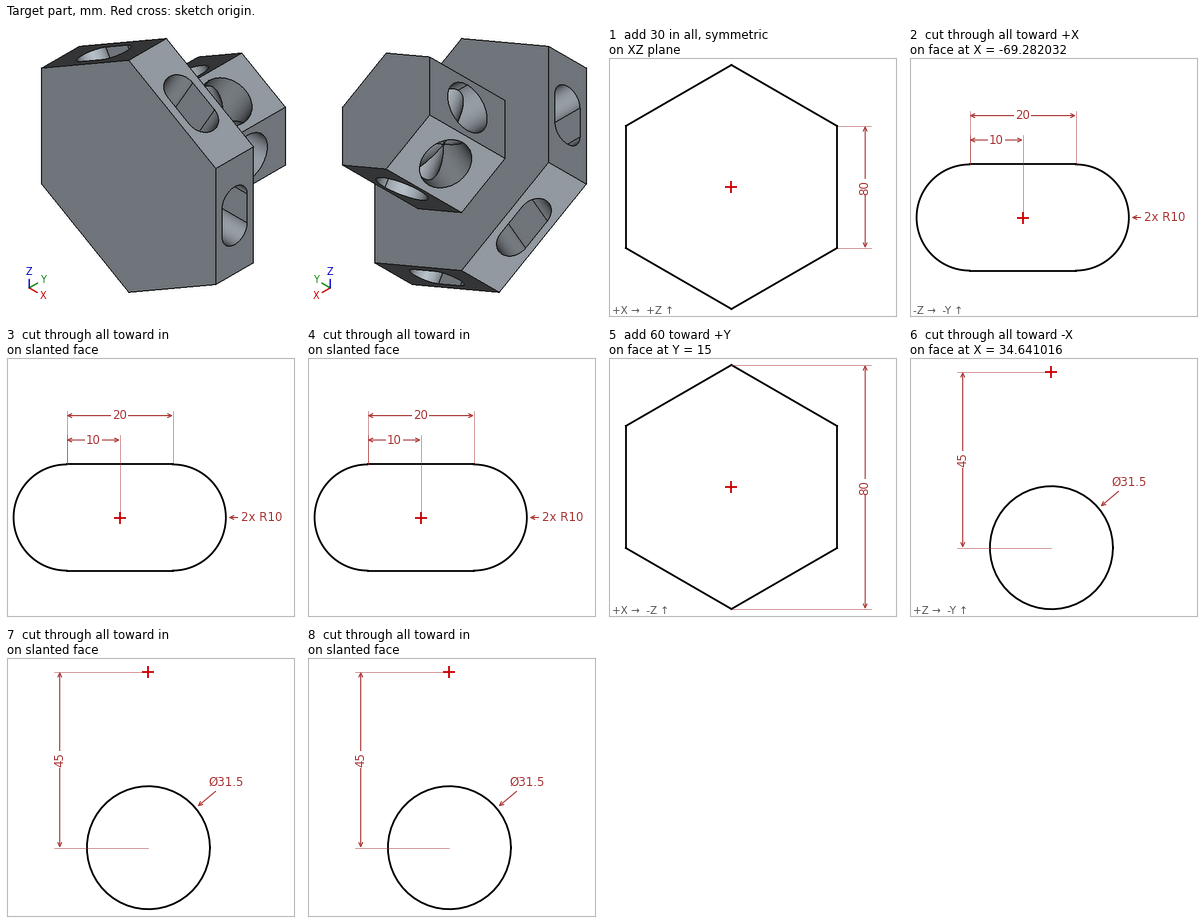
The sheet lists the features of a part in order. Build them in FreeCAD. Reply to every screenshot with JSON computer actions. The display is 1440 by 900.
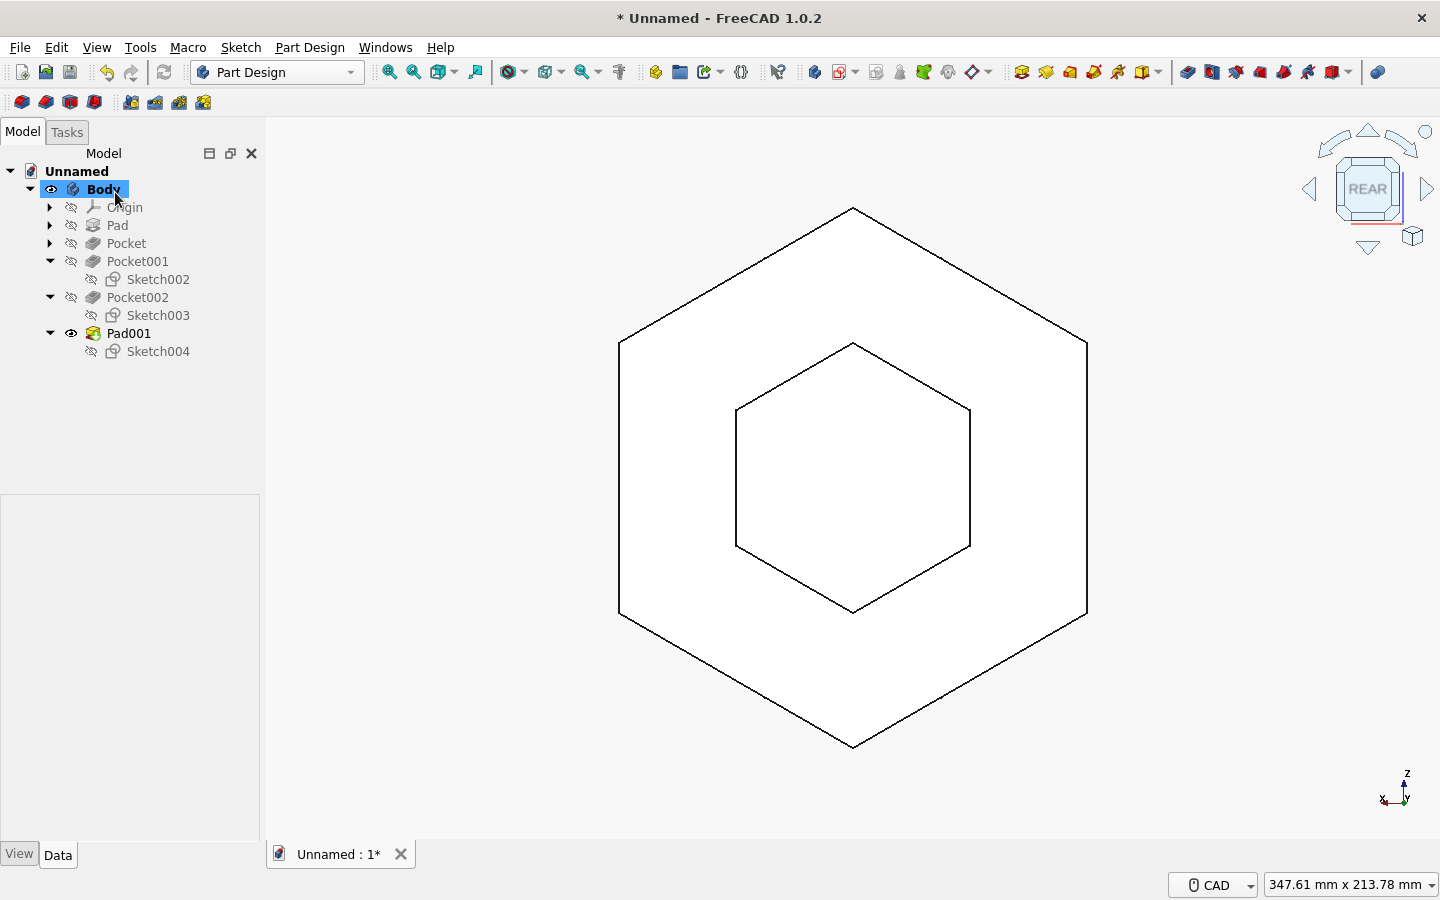
{"action": "key", "text": "0"}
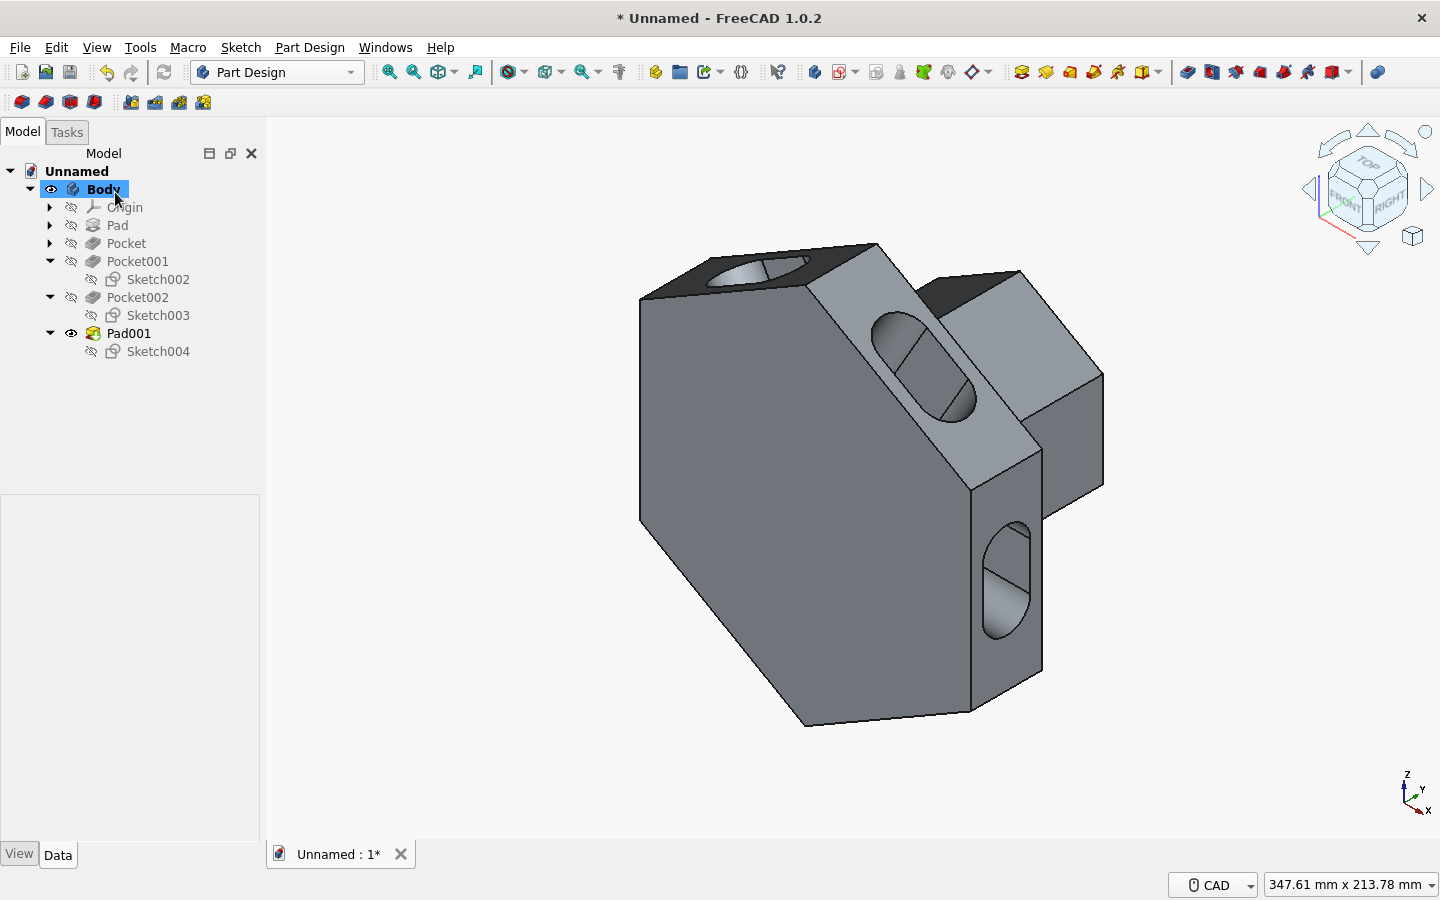
{"action": "left_click", "coordinate": [390, 72]}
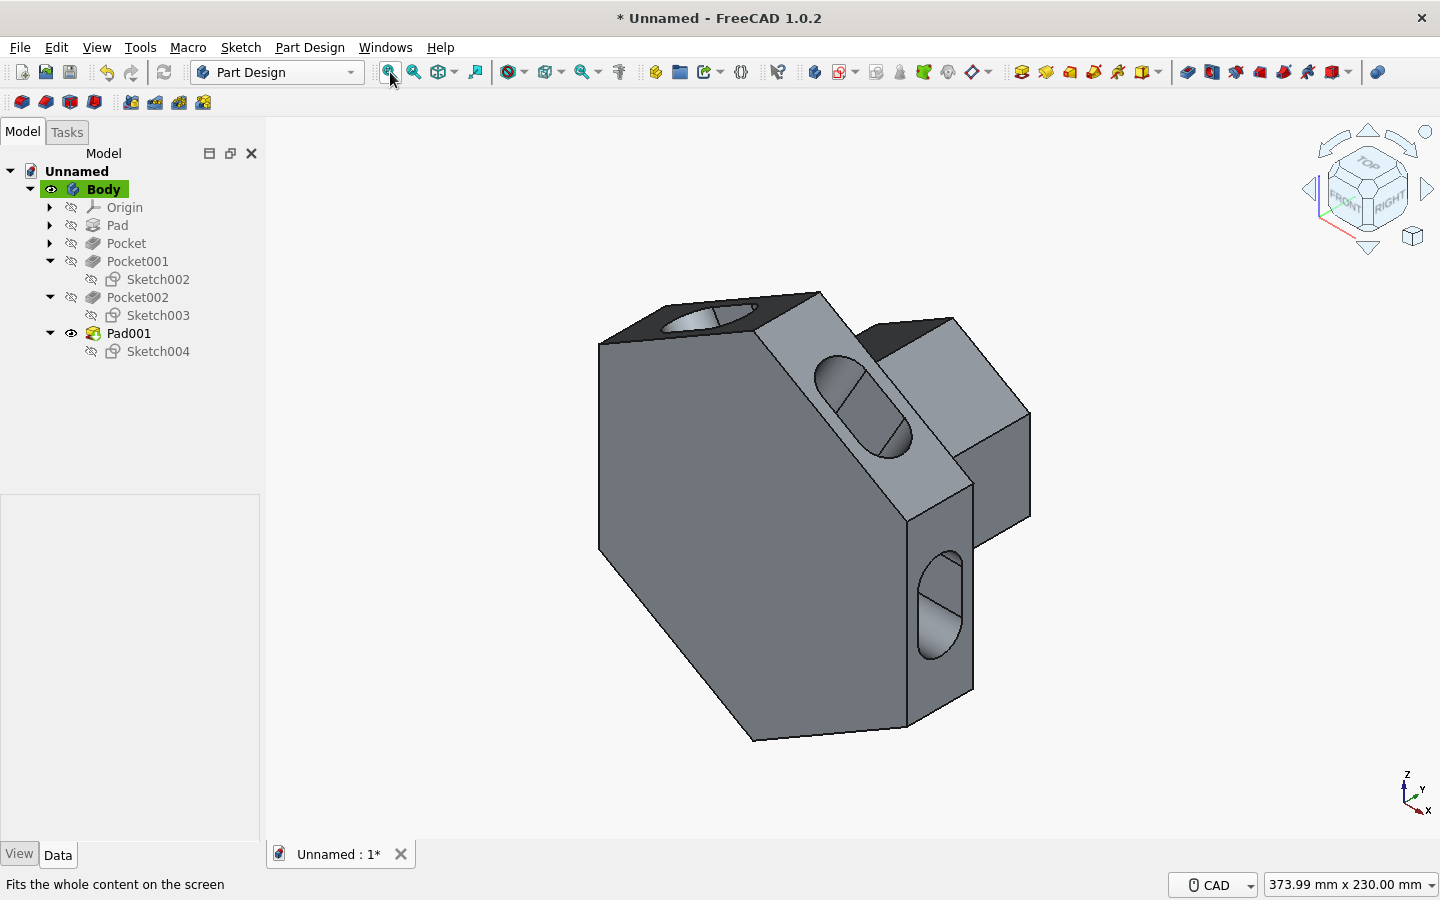
{"action": "left_click", "coordinate": [982, 491]}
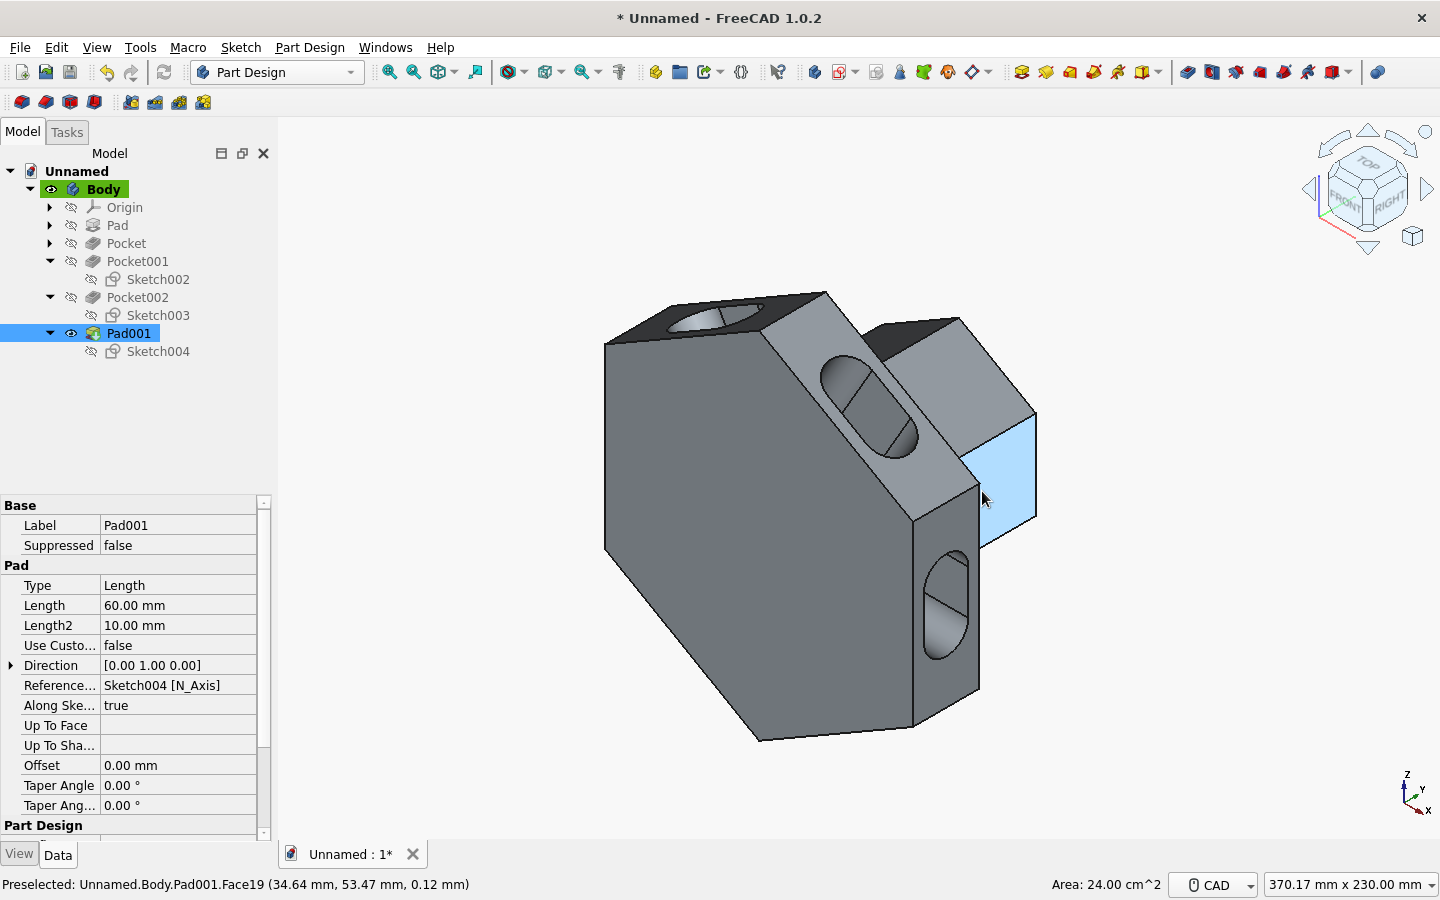
{"action": "left_click", "coordinate": [840, 72]}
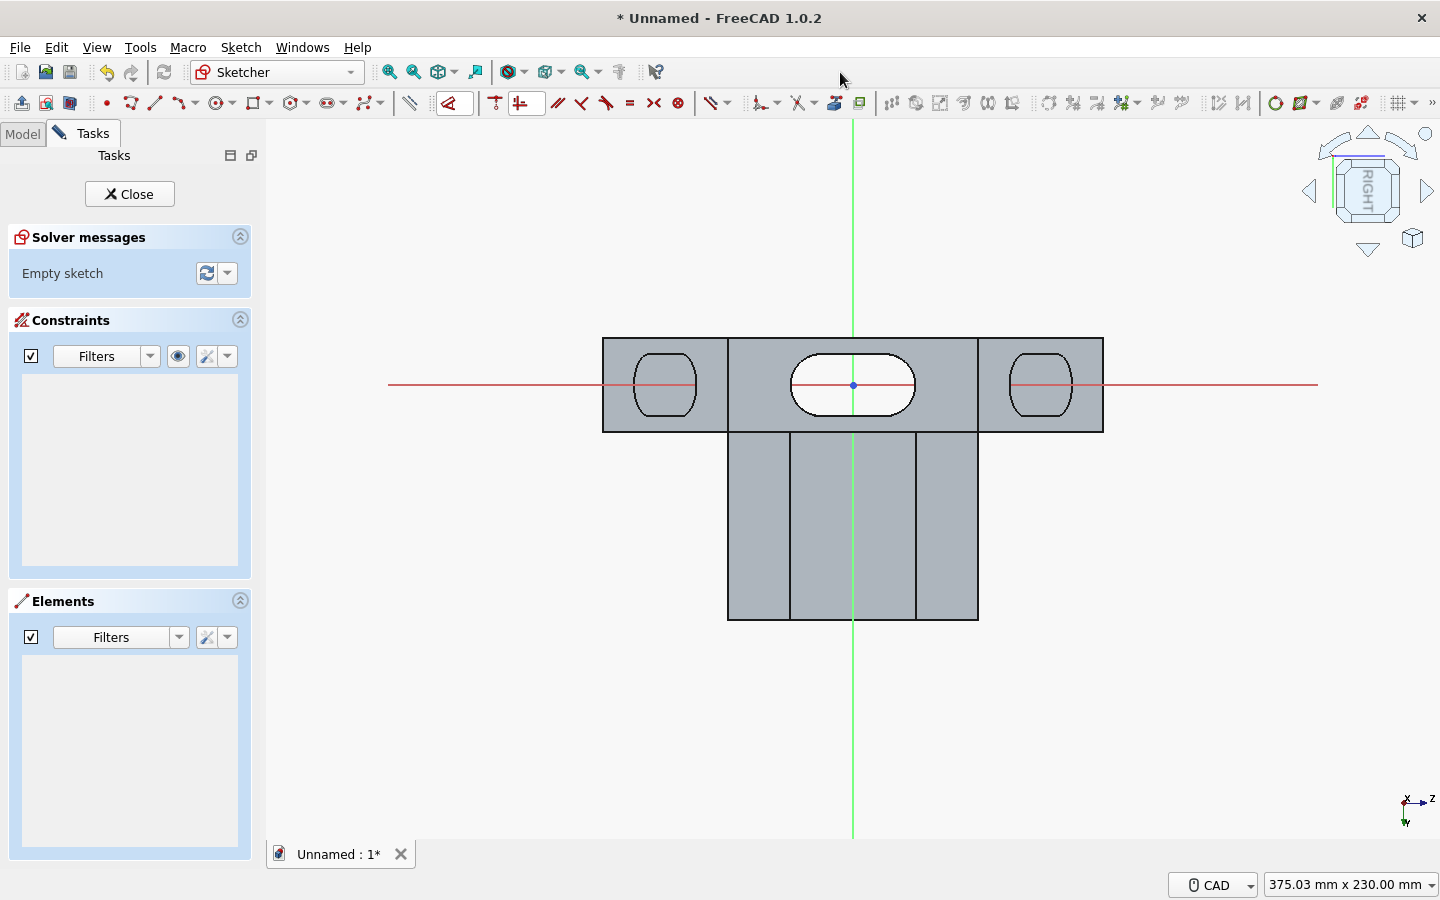
{"action": "left_click", "coordinate": [70, 104]}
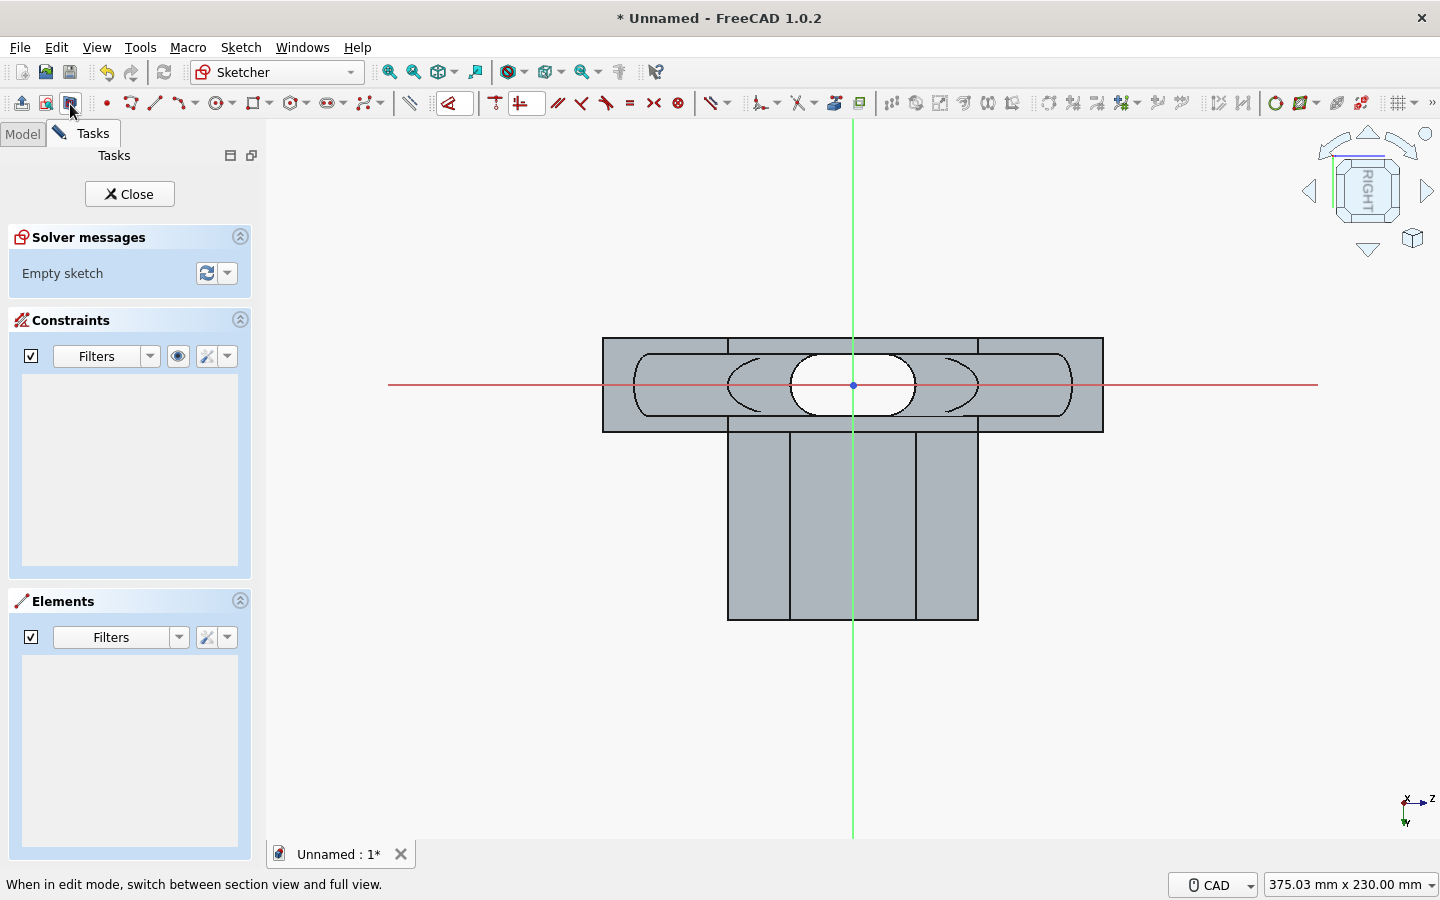
{"action": "scroll", "coordinate": [893, 481], "scroll_direction": "up", "scroll_amount": 5}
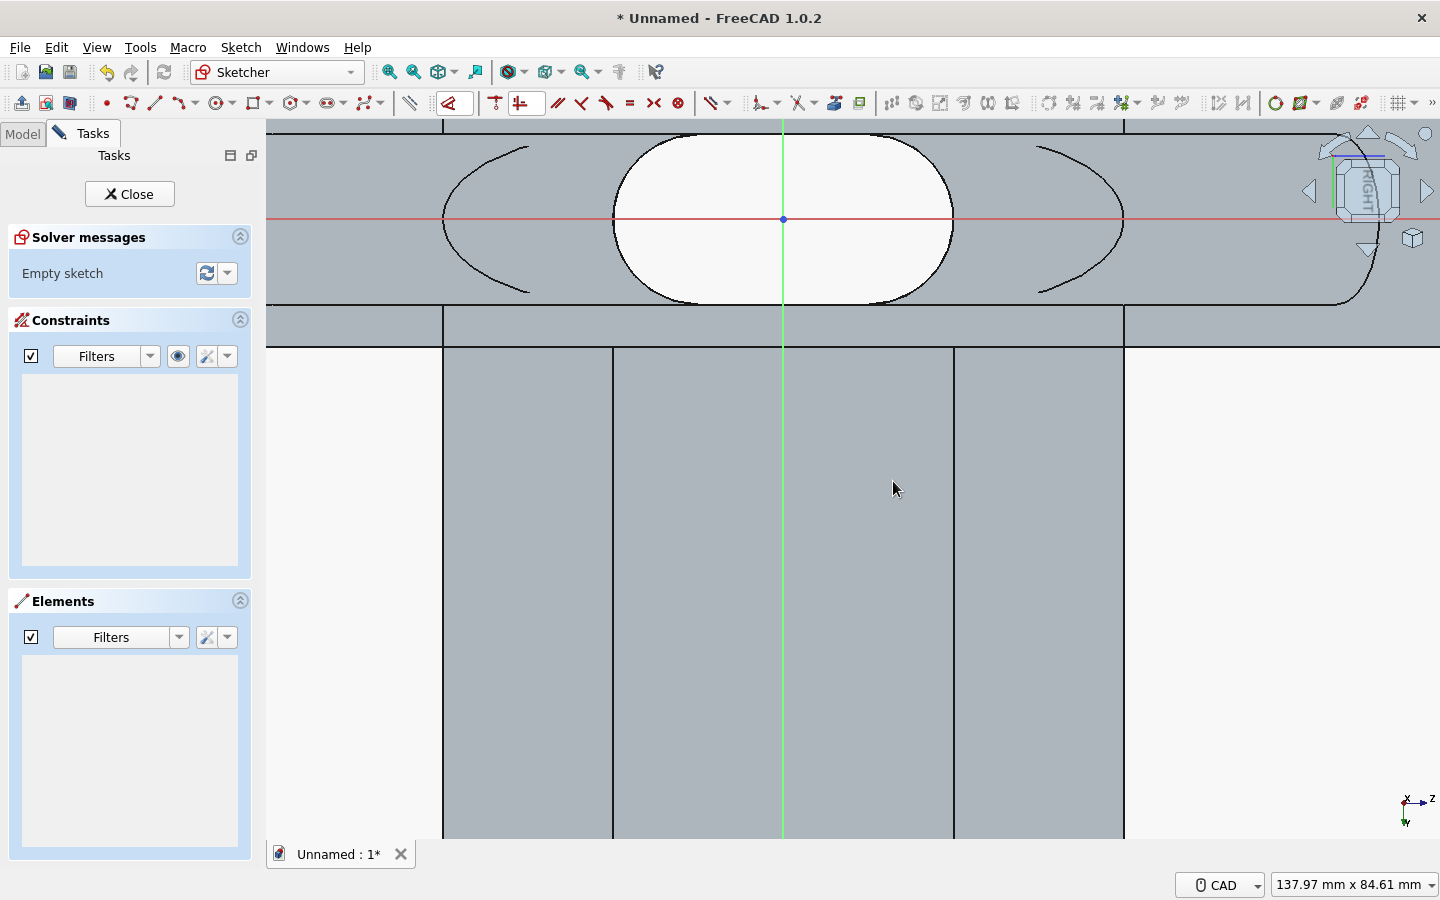
{"action": "left_click", "coordinate": [216, 104]}